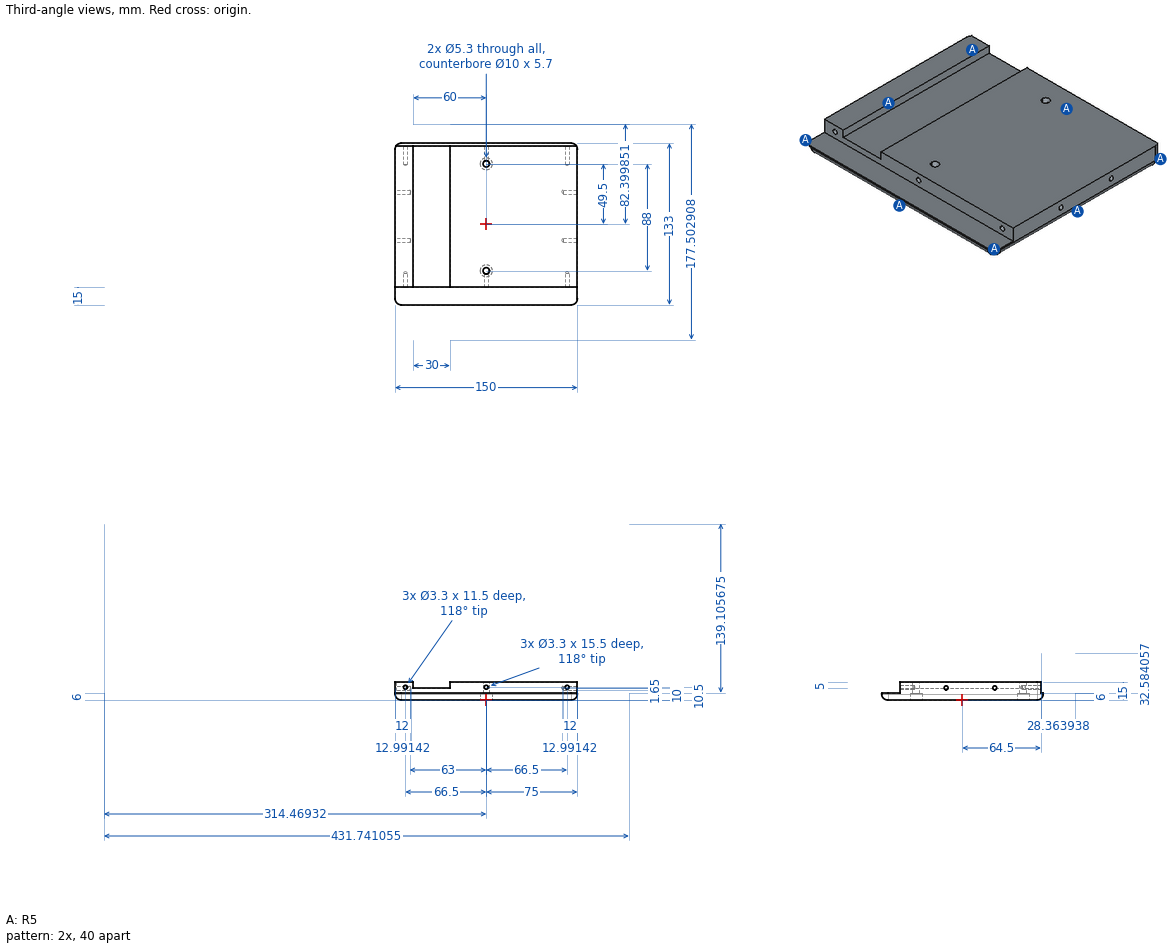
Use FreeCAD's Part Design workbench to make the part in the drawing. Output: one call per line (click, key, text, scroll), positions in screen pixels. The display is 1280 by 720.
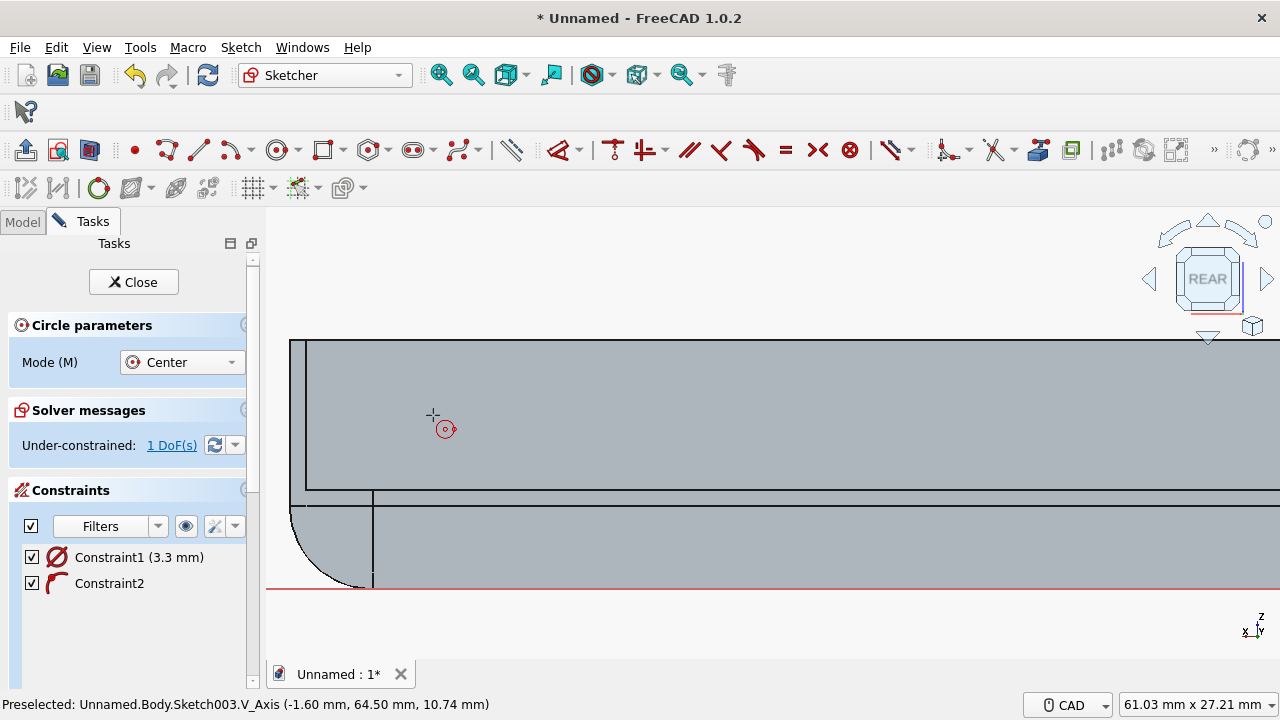
scroll(432, 415, down, 7)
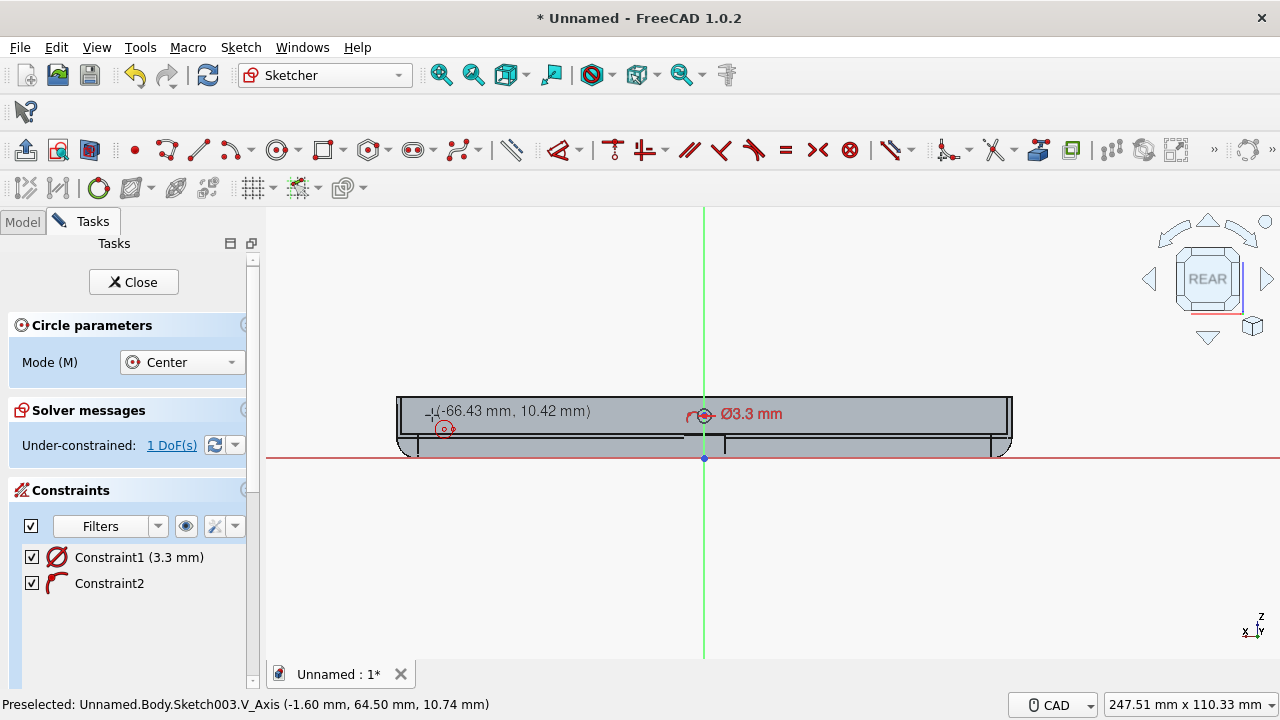
click(432, 415)
move(437, 411)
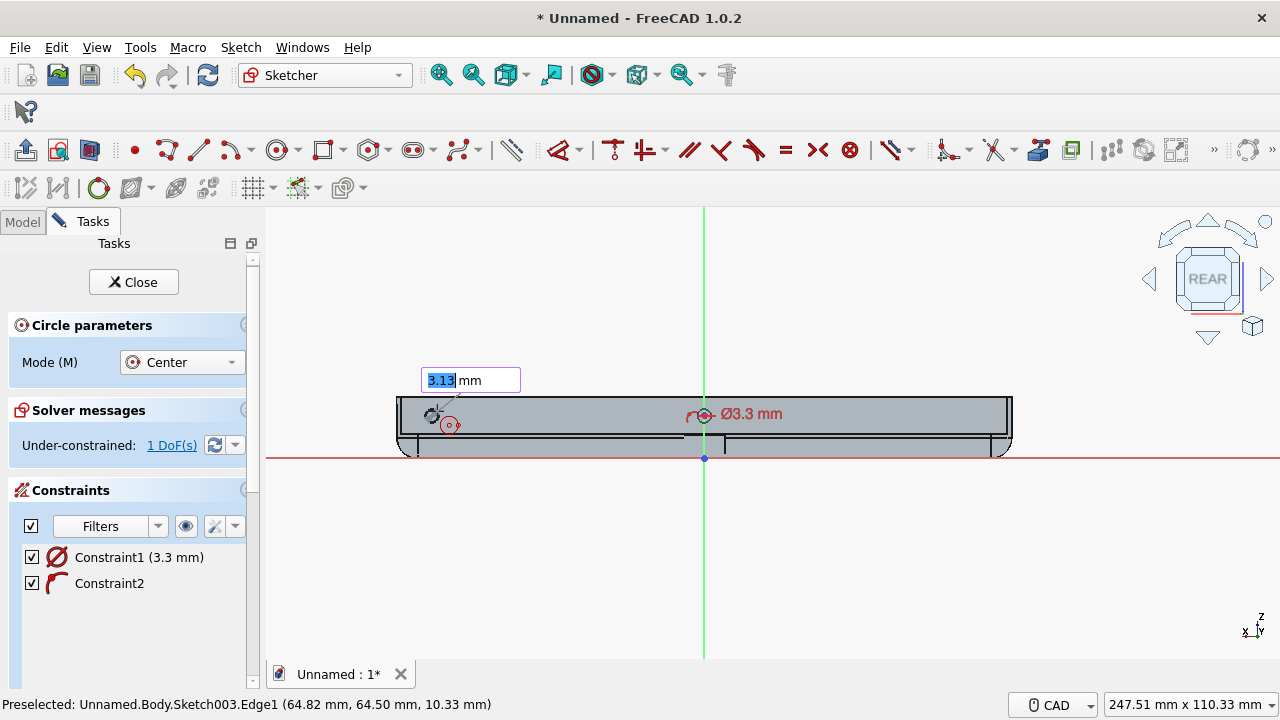
text(3.3)
key(Return)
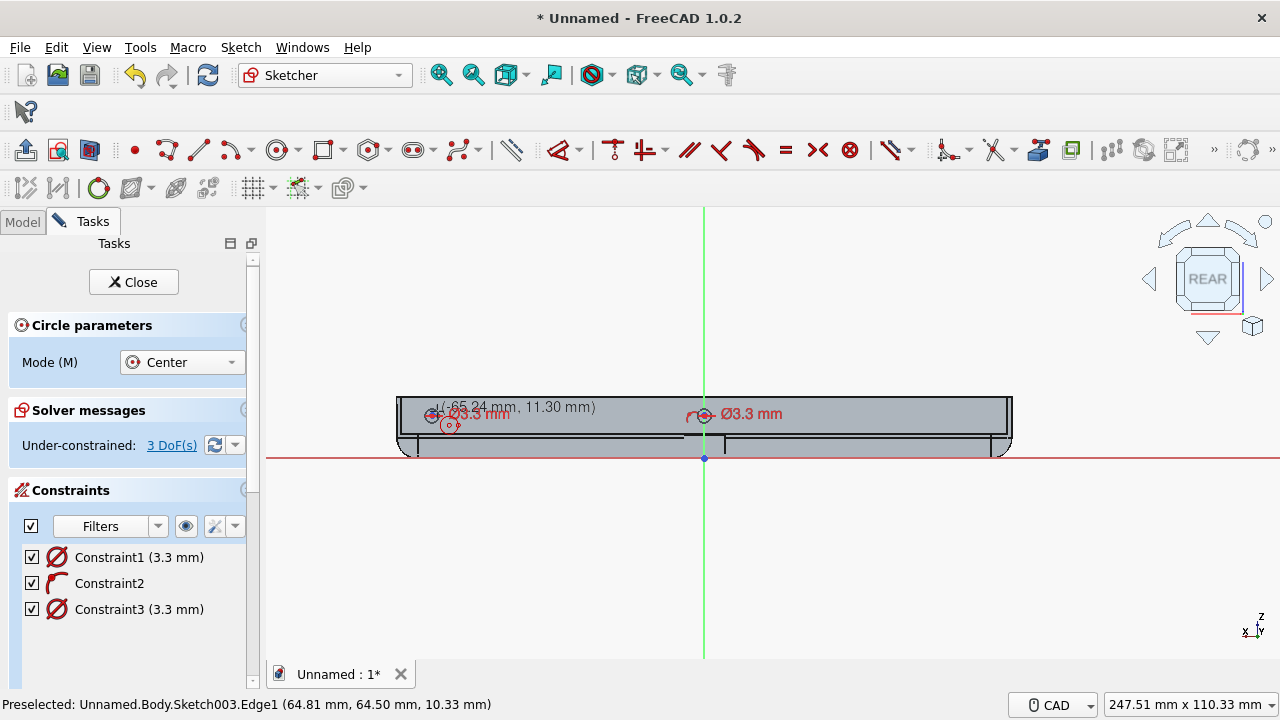
scroll(977, 415, up, 7)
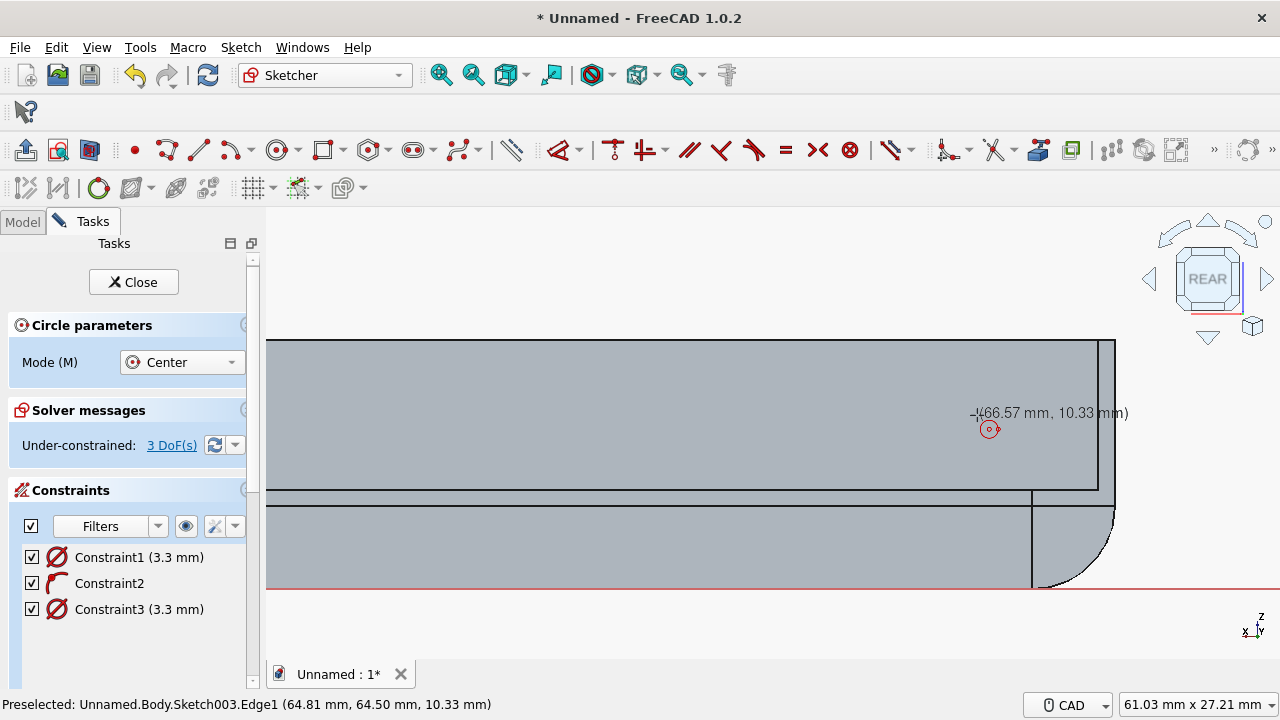
scroll(978, 415, down, 7)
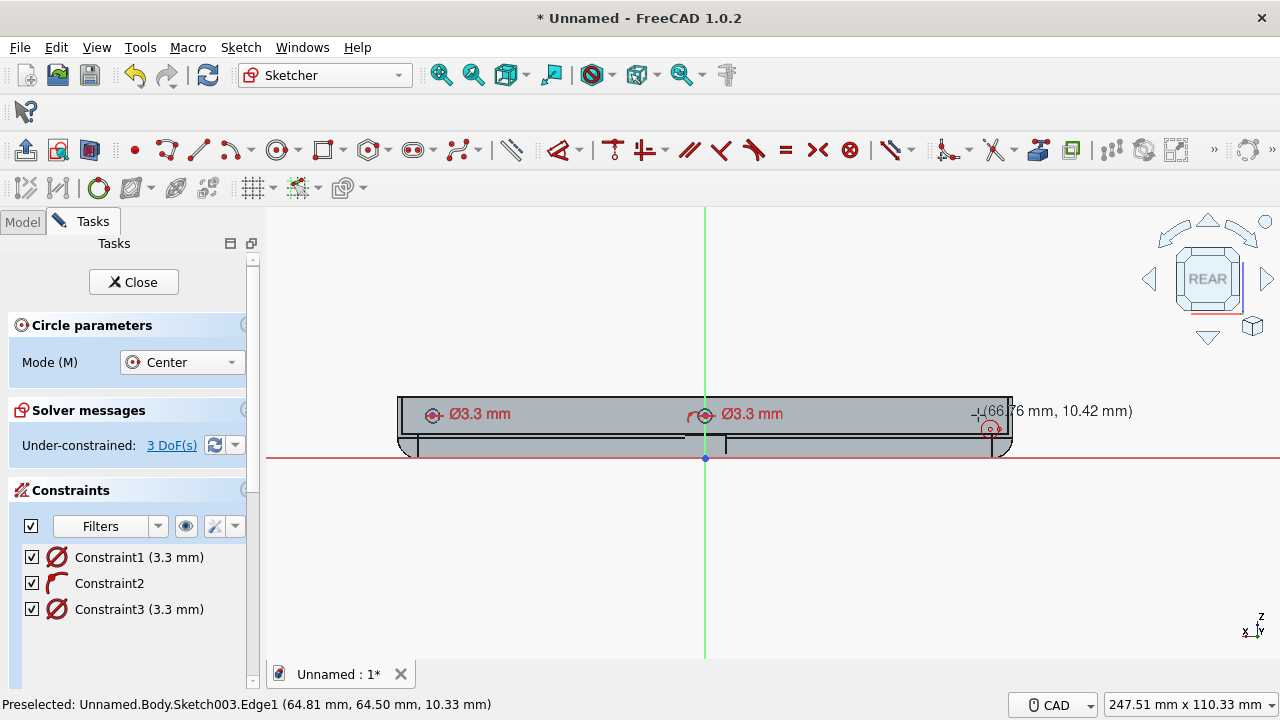
click(977, 415)
move(982, 411)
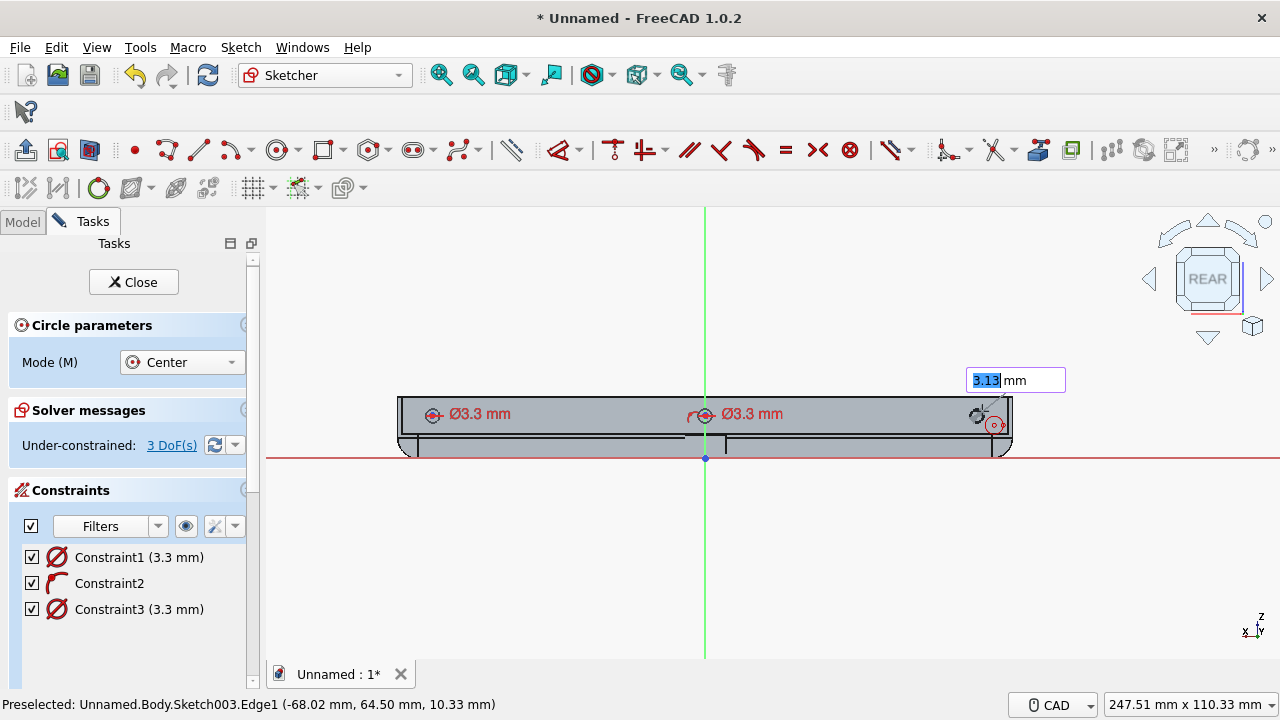
text(3.3)
key(Return)
key(Escape)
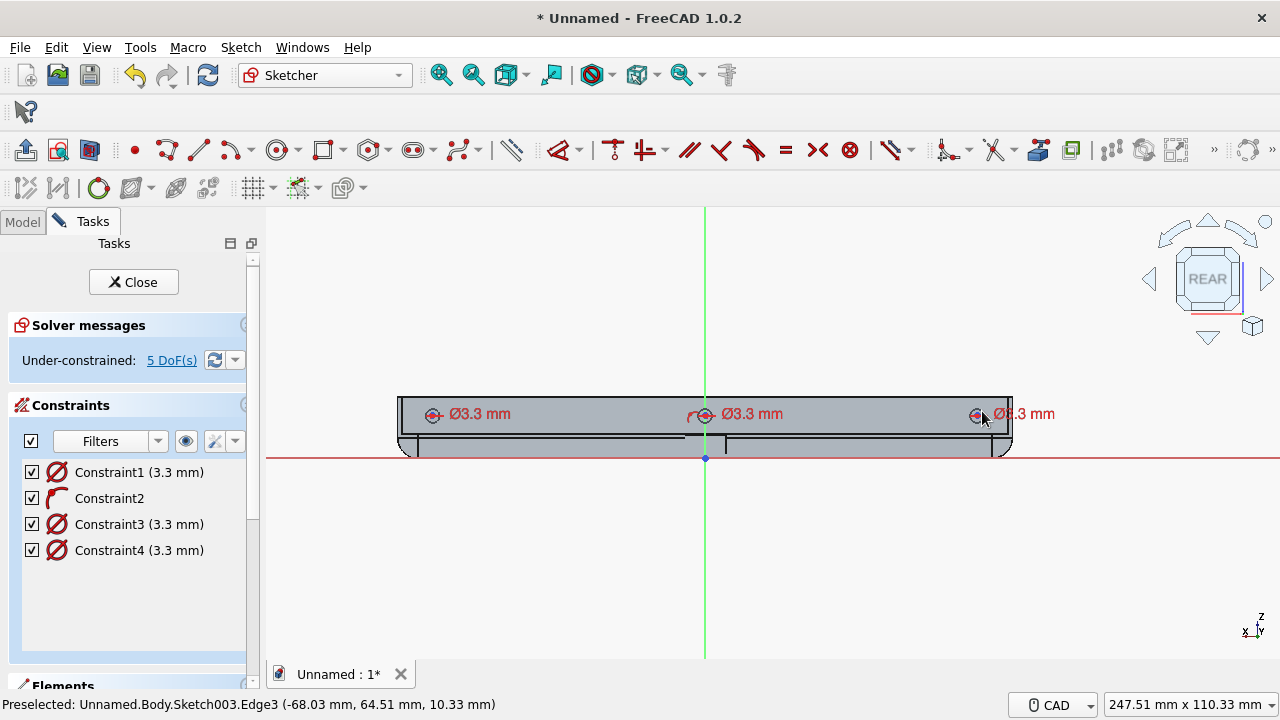
click(705, 416)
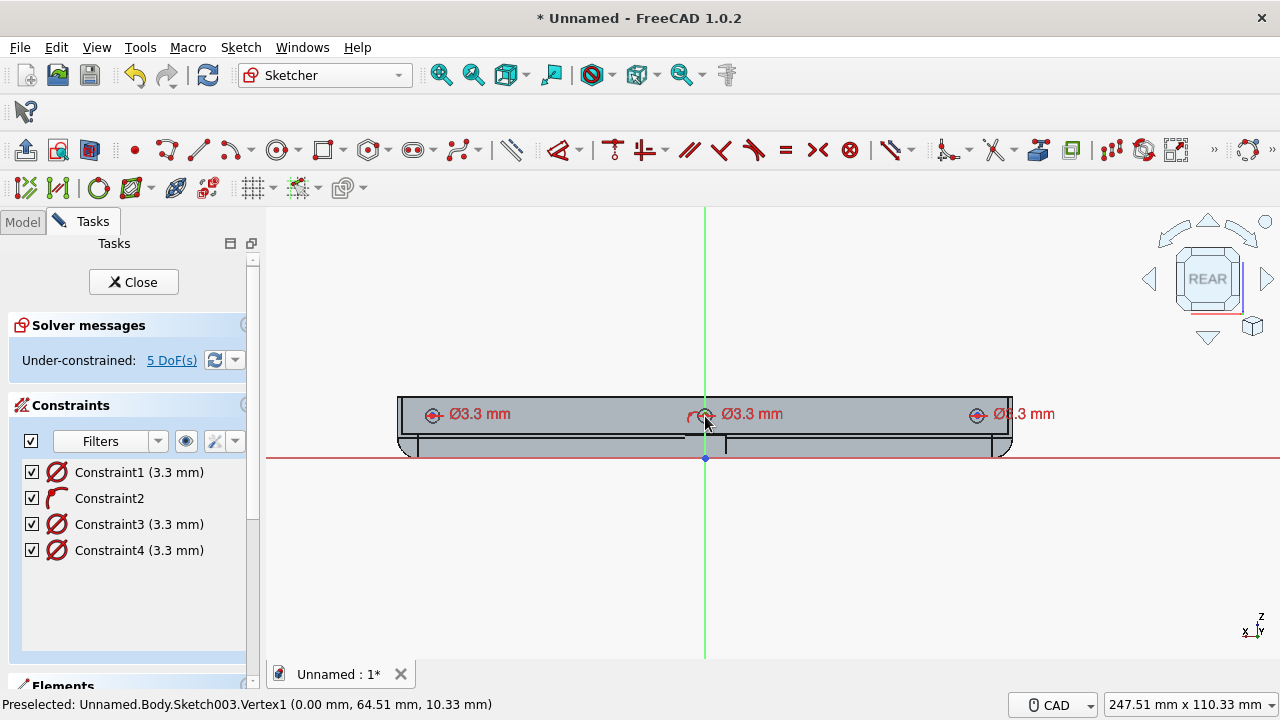
click(433, 416)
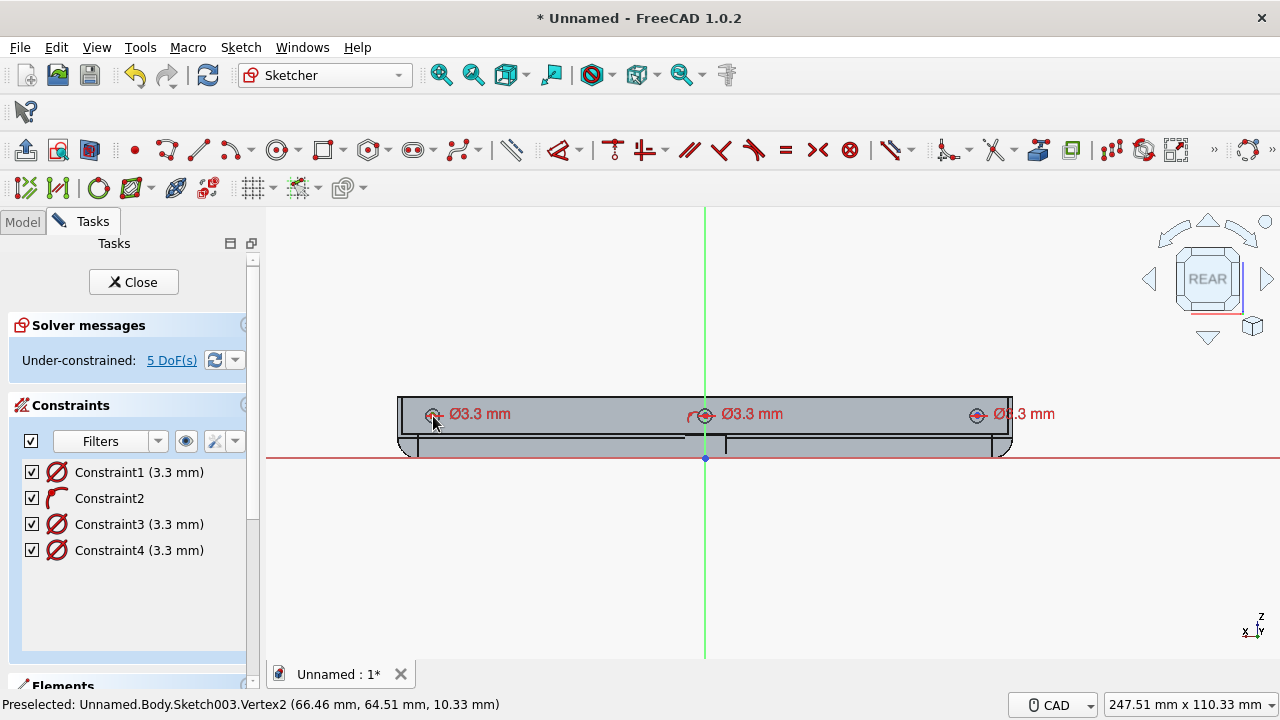
key(h)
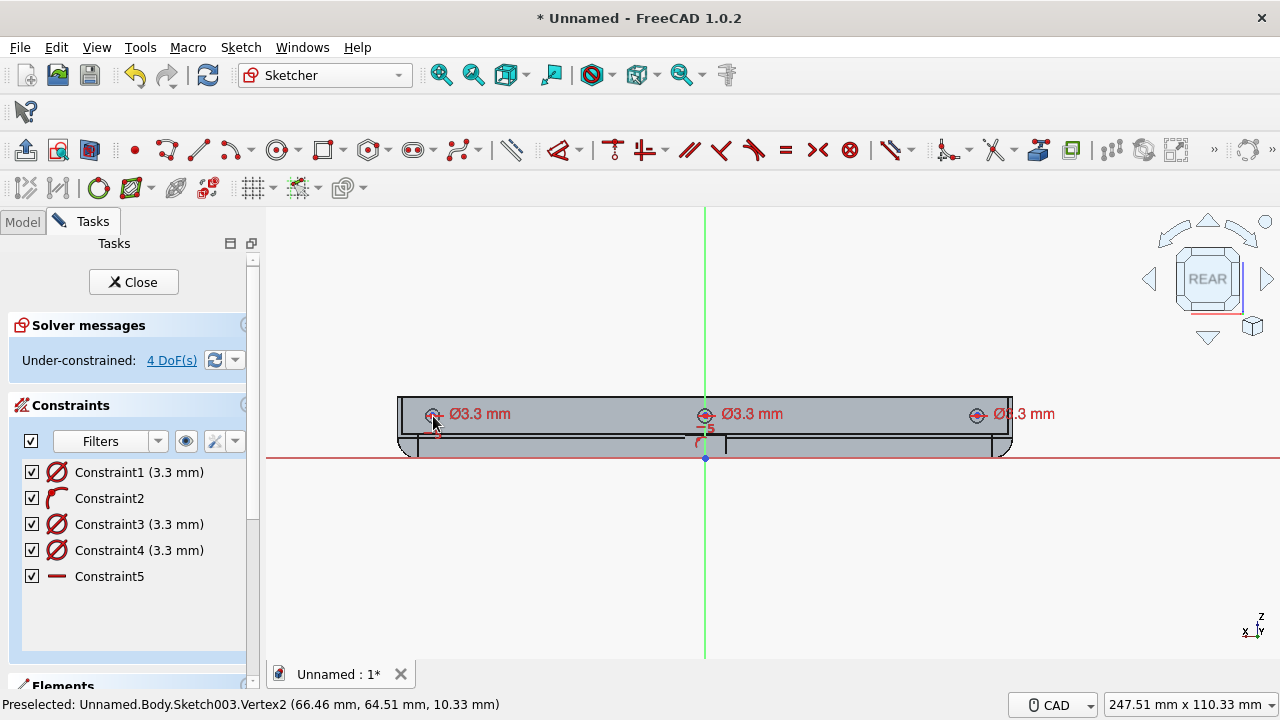
click(705, 416)